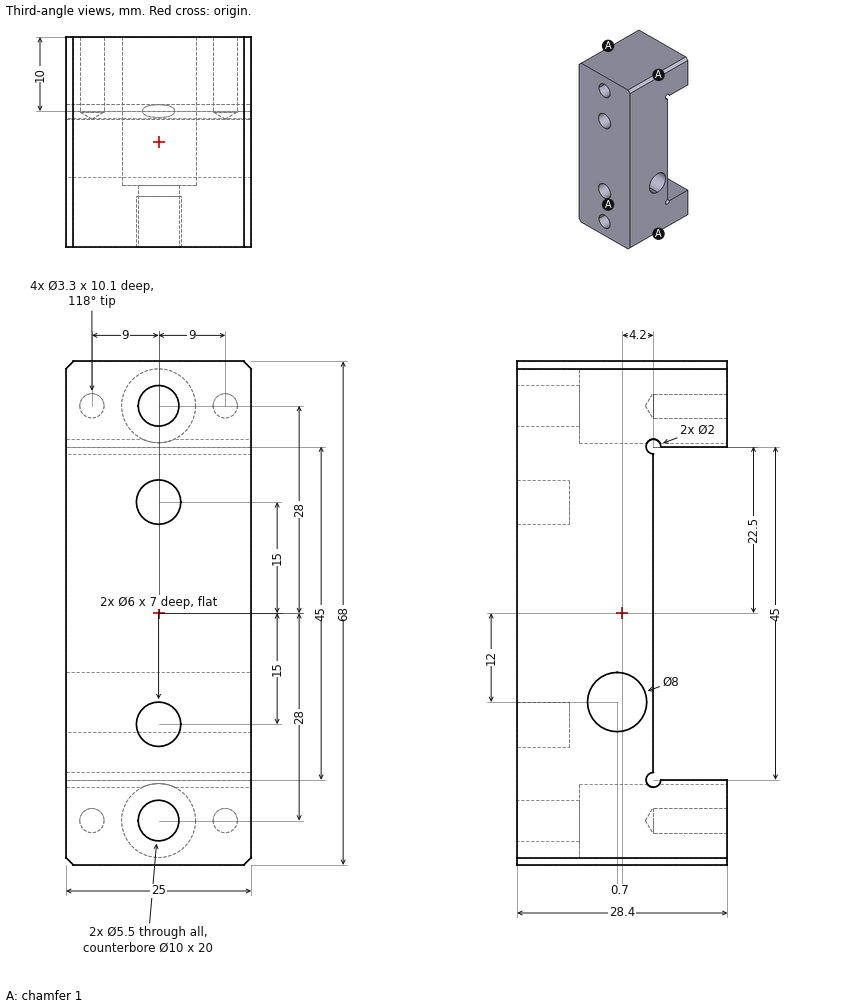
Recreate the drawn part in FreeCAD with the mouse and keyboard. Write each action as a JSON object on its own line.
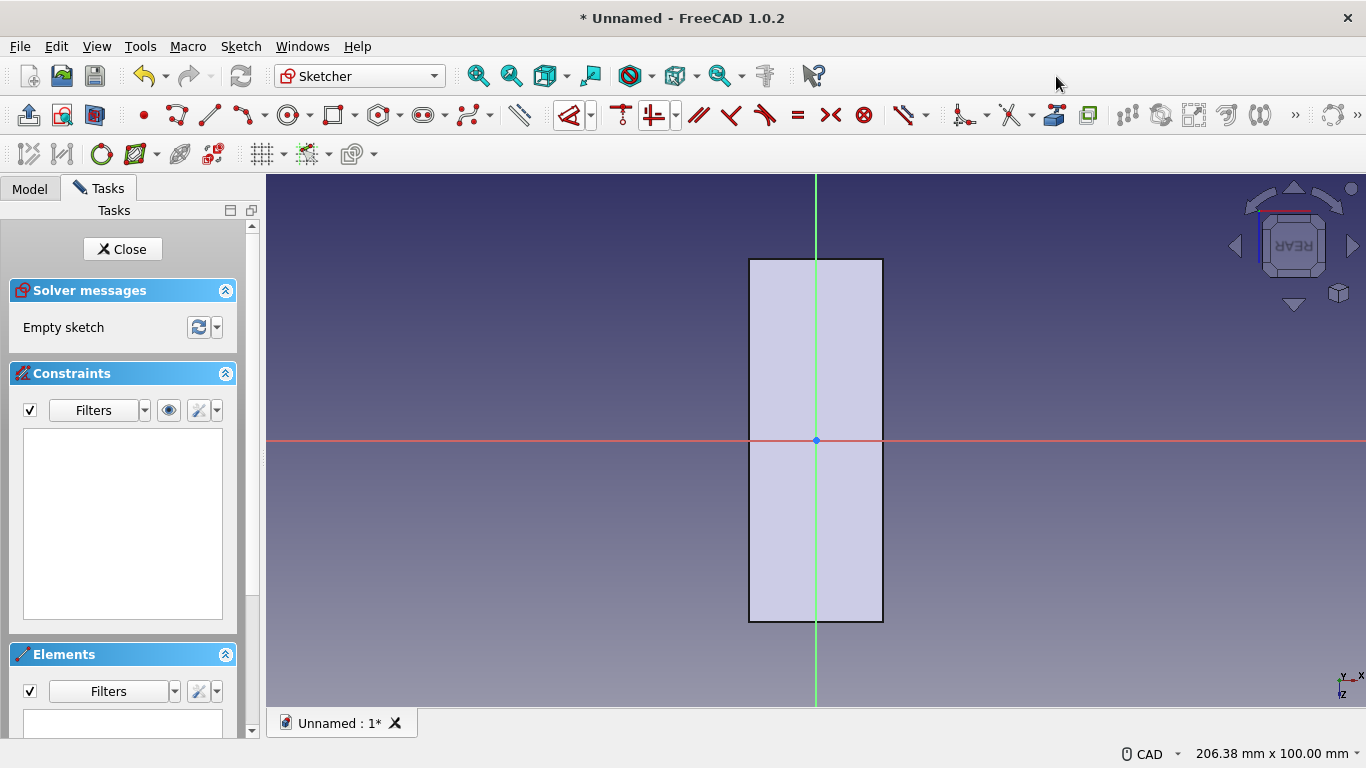
{"action": "scroll", "coordinate": [955, 441], "scroll_direction": "up", "scroll_amount": 2}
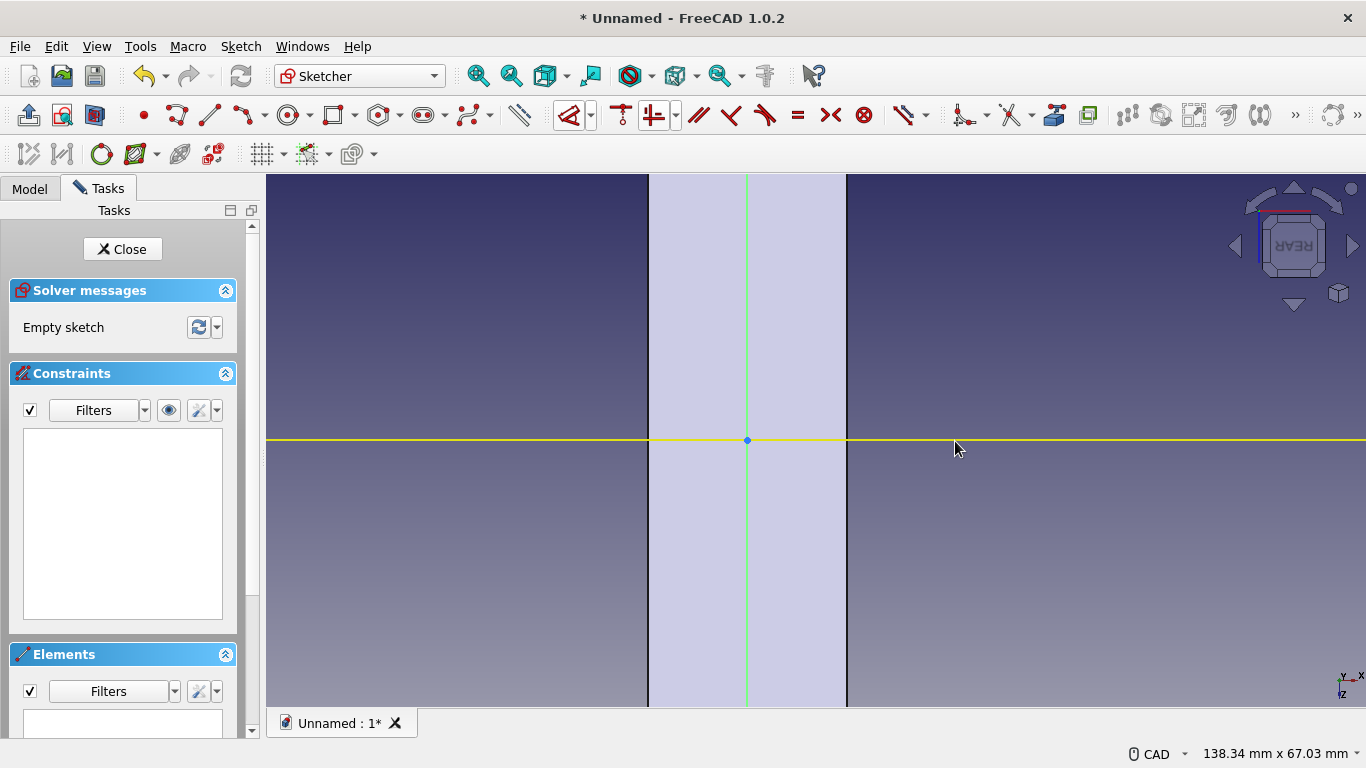
{"action": "key", "text": "g v"}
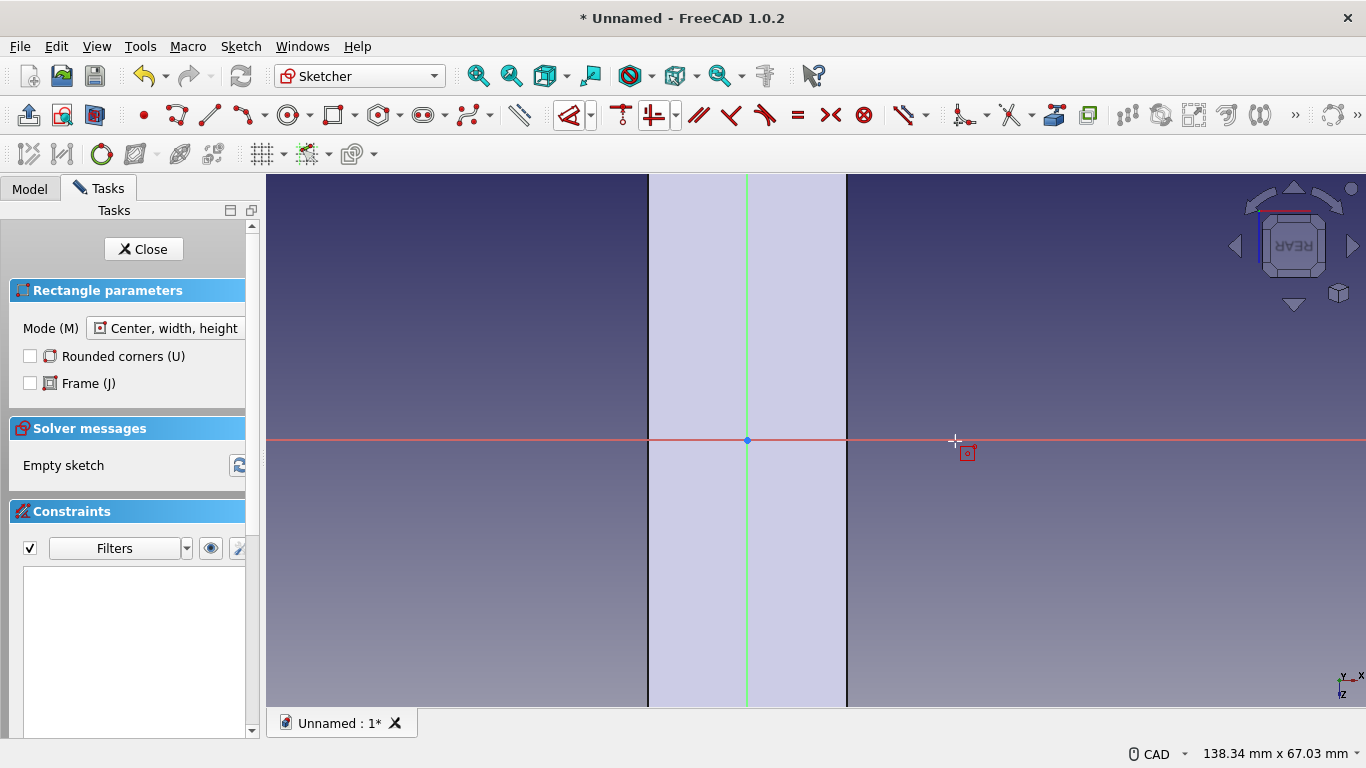
{"action": "left_click", "coordinate": [747, 440]}
{"action": "left_click", "coordinate": [847, 261]}
{"action": "key", "text": "Escape"}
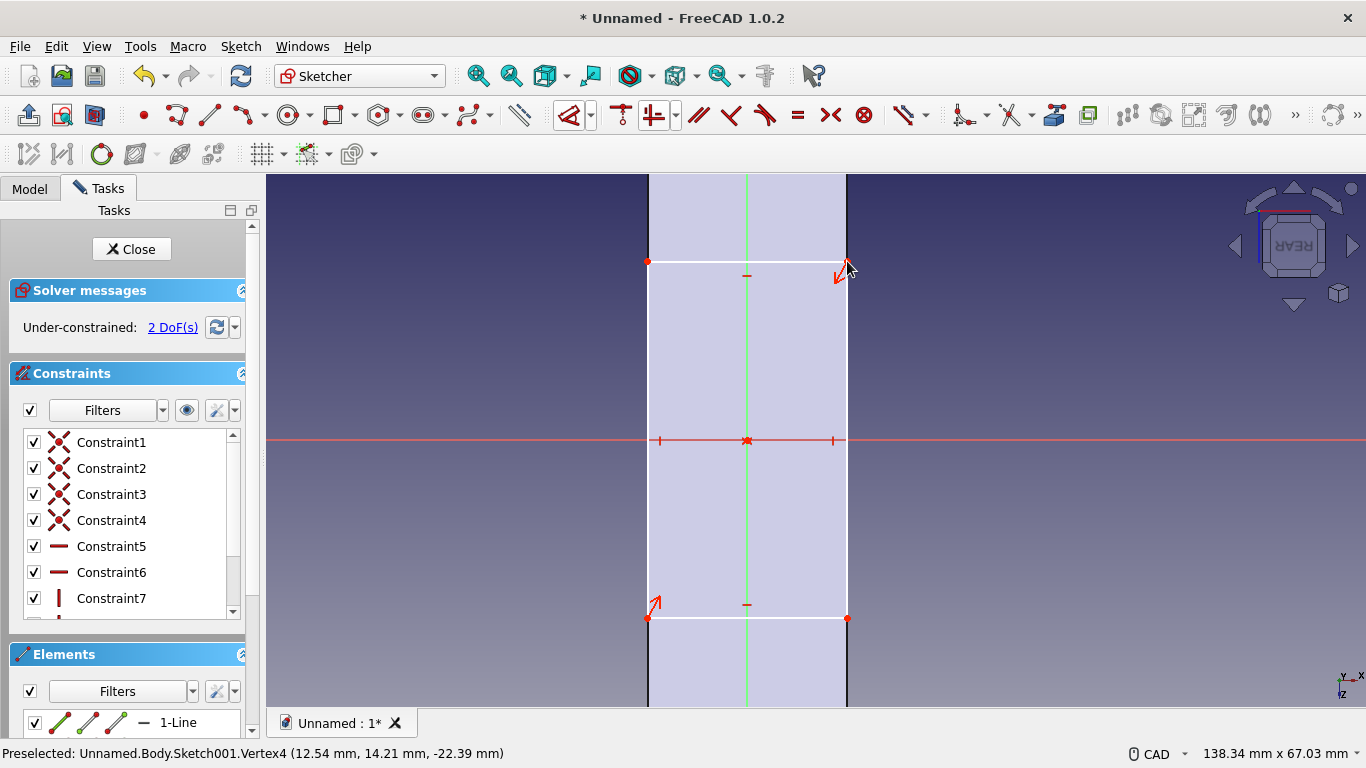
{"action": "left_click", "coordinate": [568, 116]}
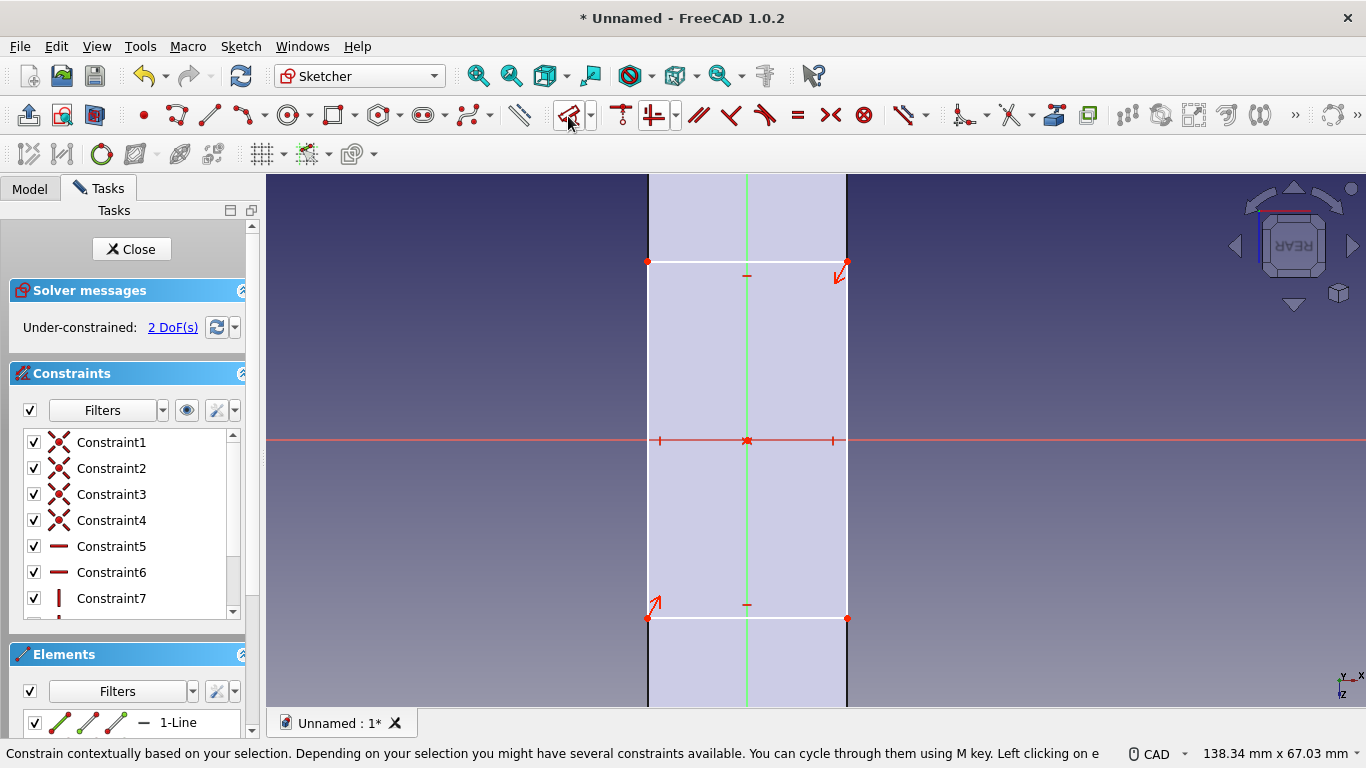
{"action": "left_click", "coordinate": [707, 618]}
{"action": "left_click", "coordinate": [701, 652]}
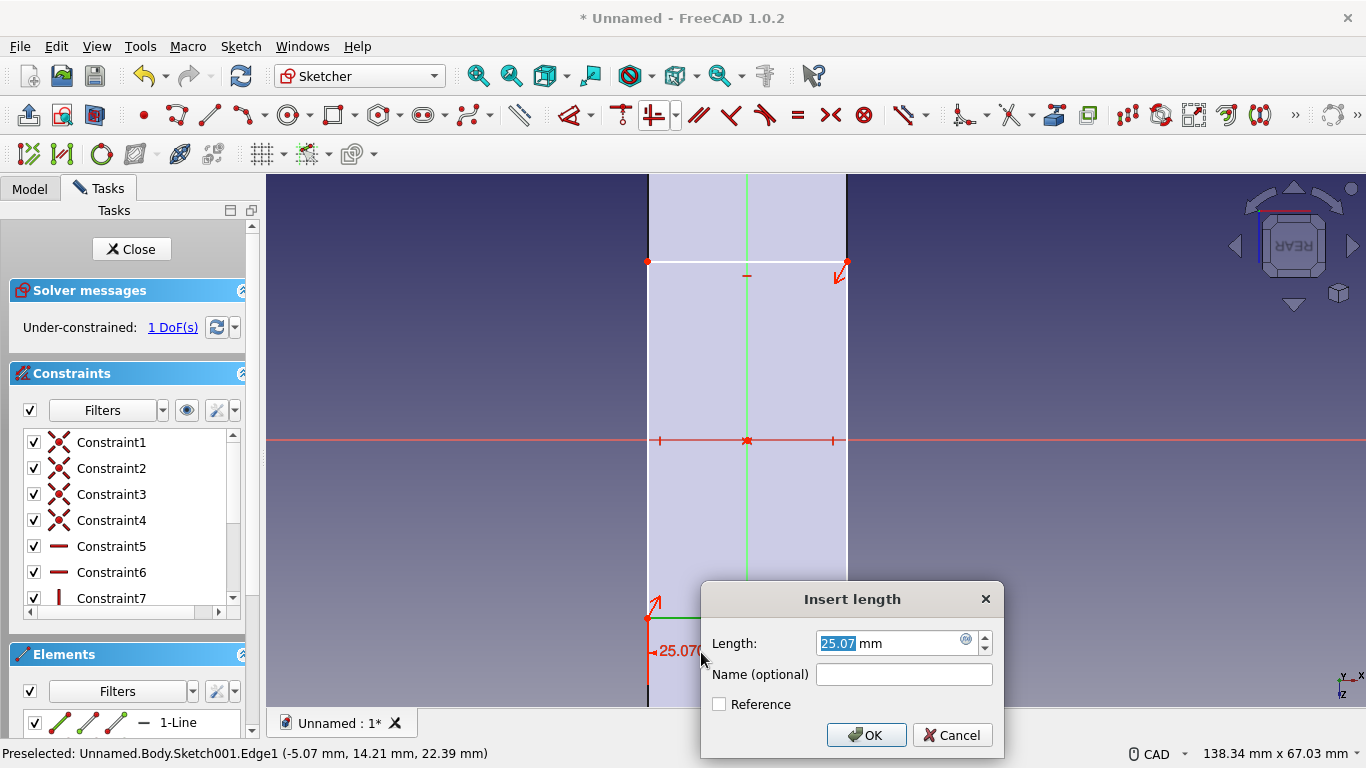
{"action": "type", "text": "25"}
{"action": "key", "text": "Return"}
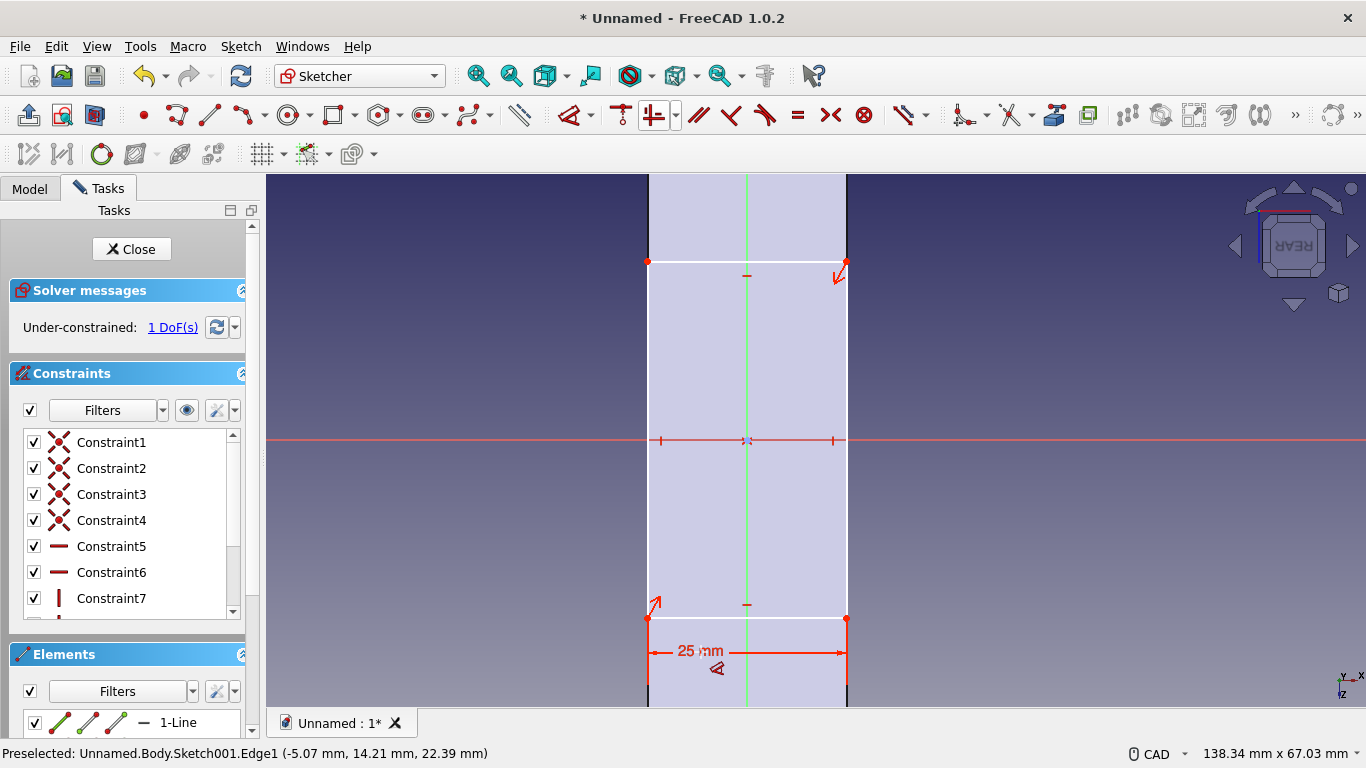
{"action": "left_click", "coordinate": [847, 511]}
{"action": "left_click", "coordinate": [881, 358]}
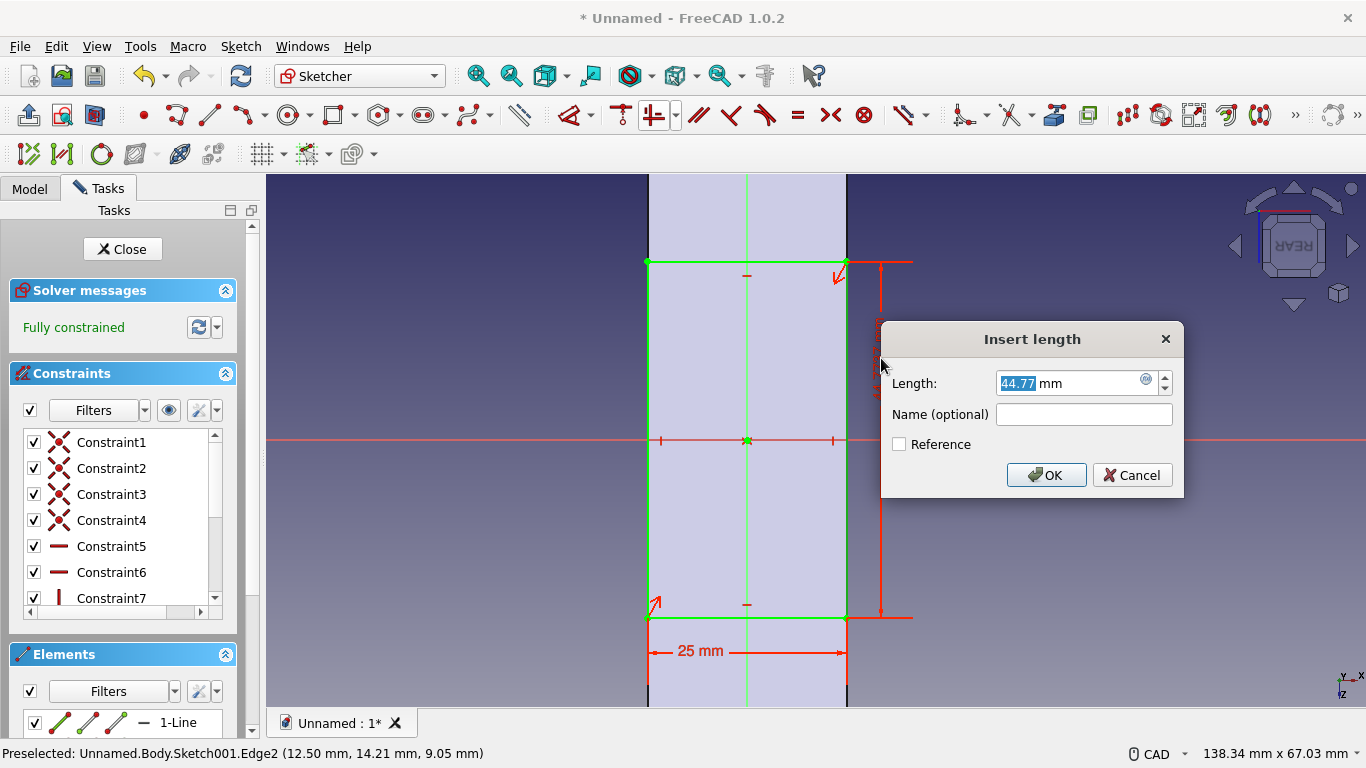
{"action": "type", "text": "45"}
{"action": "key", "text": "Return"}
{"action": "key", "text": "Escape"}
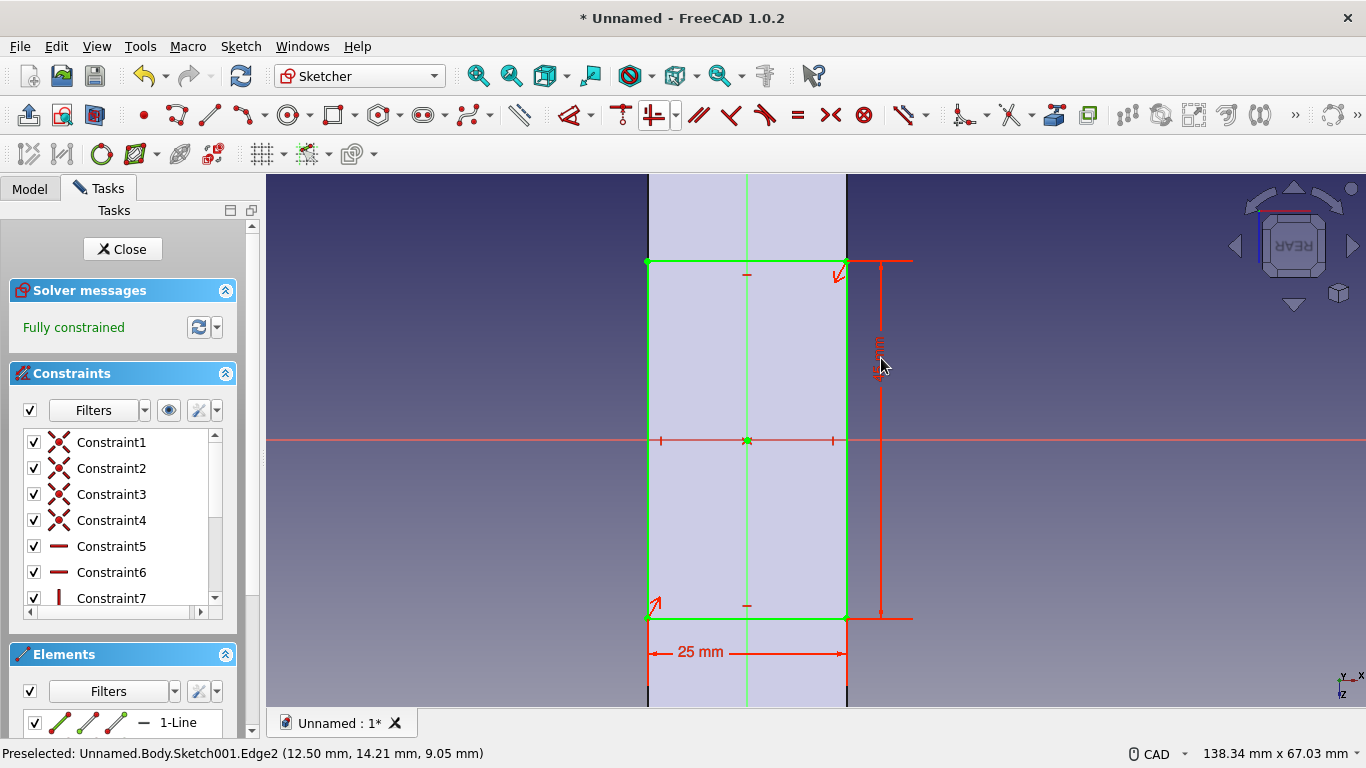
{"action": "left_click", "coordinate": [123, 249]}